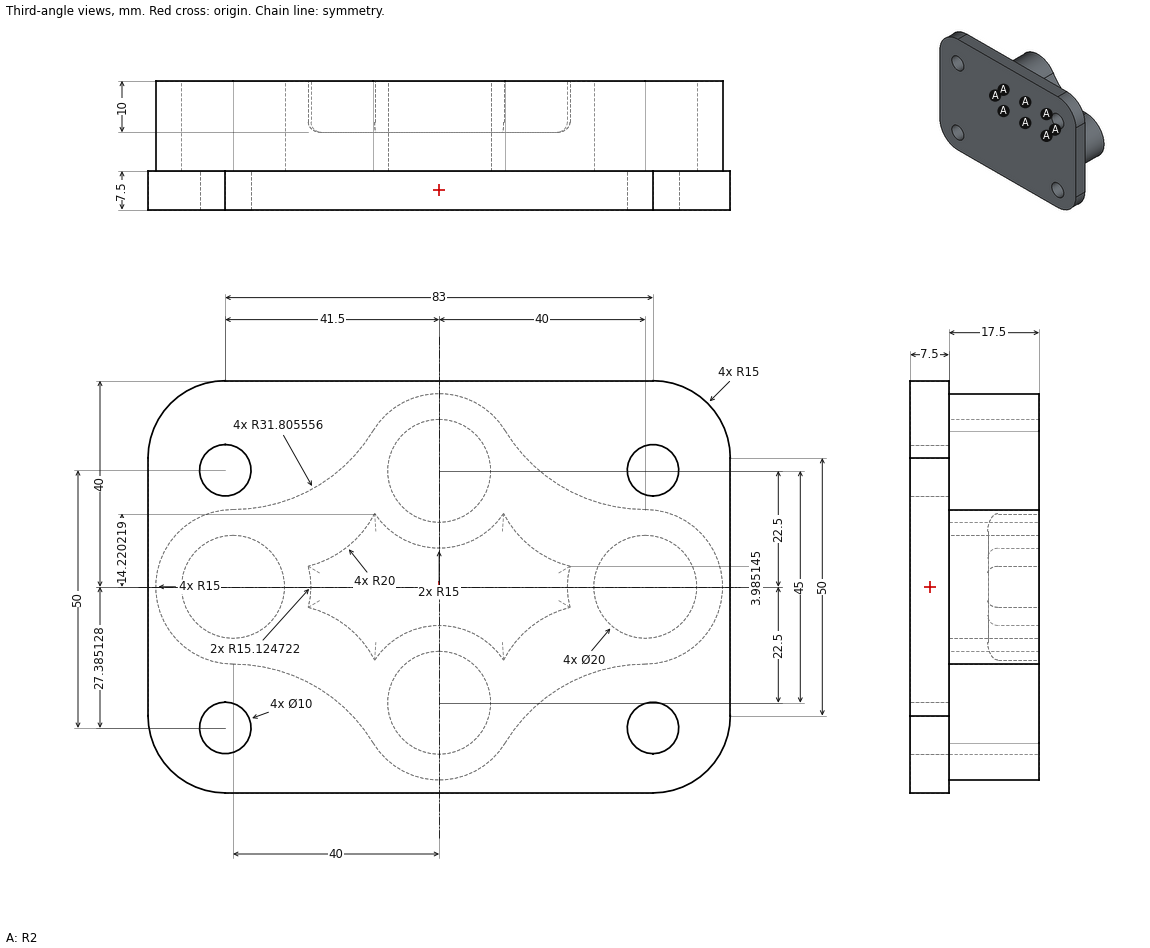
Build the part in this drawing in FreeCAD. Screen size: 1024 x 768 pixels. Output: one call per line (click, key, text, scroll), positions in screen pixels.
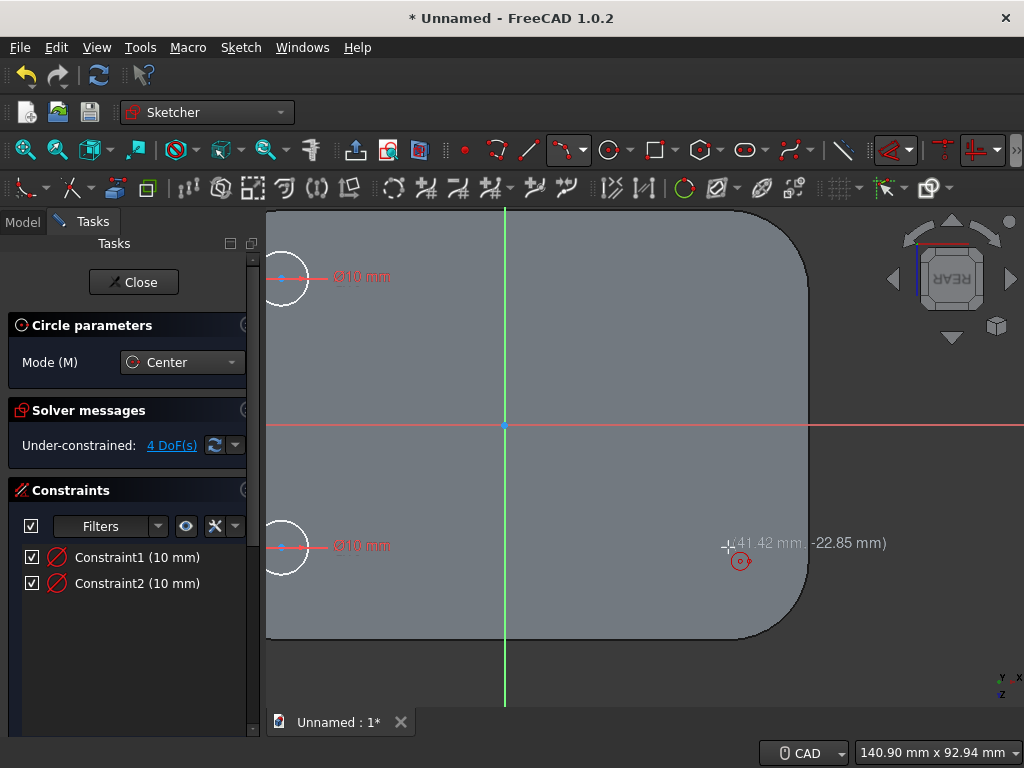
click(728, 547)
move(747, 528)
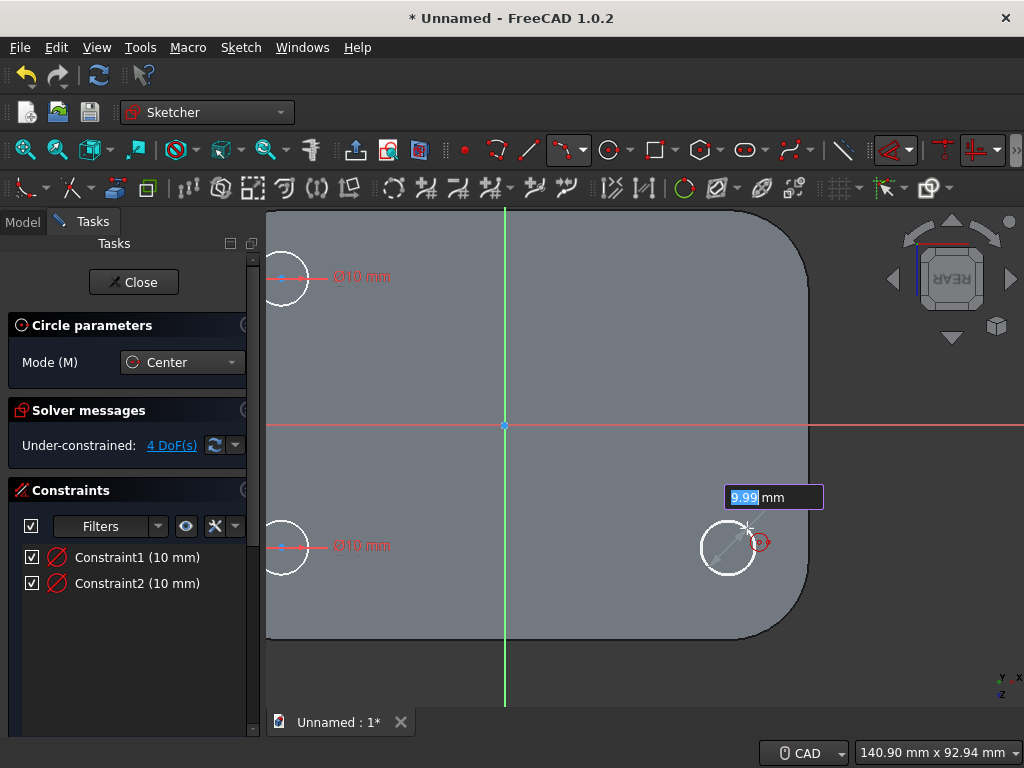
text(10)
key(Return)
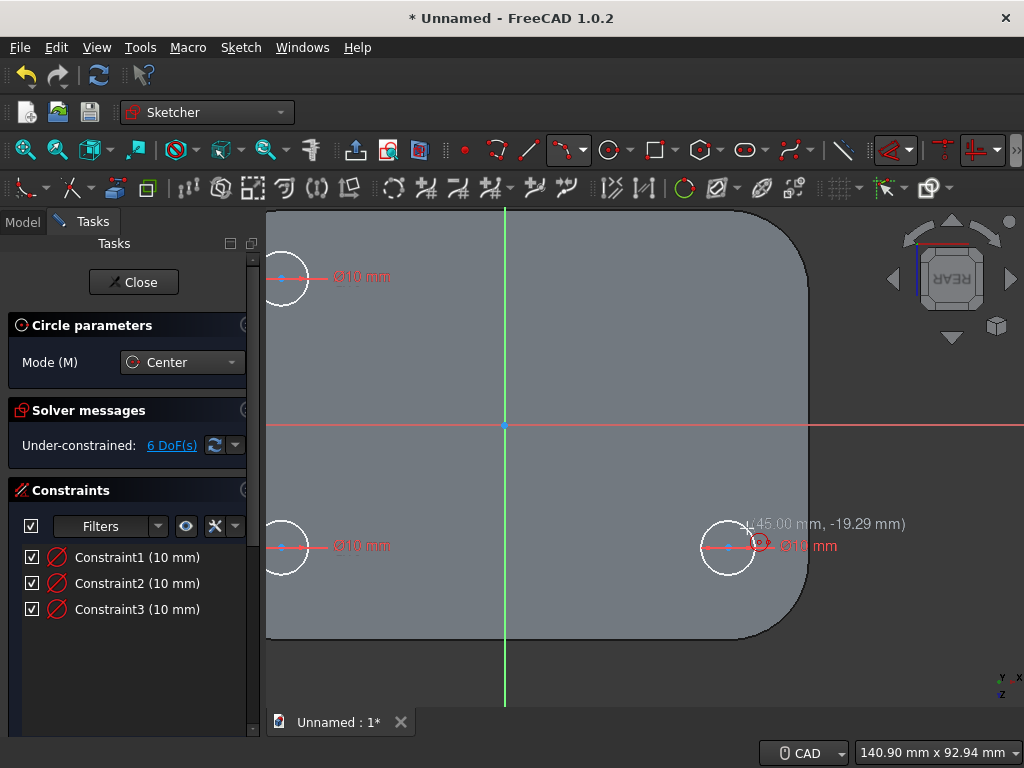
click(728, 278)
move(747, 259)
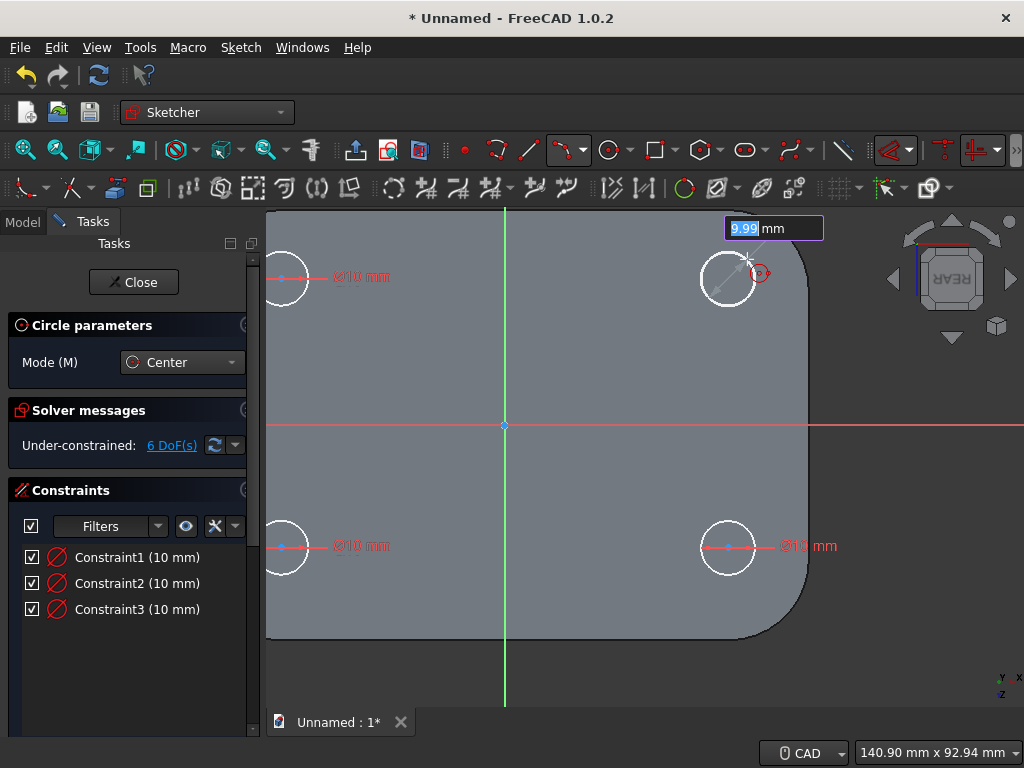
text(10)
key(Return)
key(Escape)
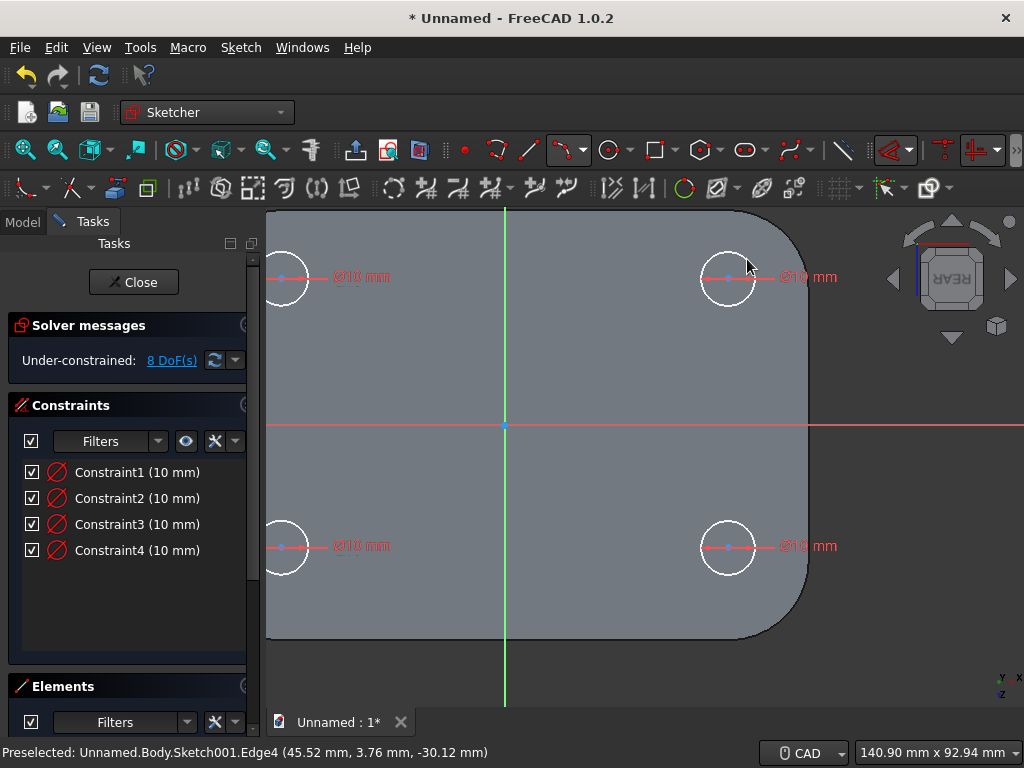
scroll(859, 659, down, 1)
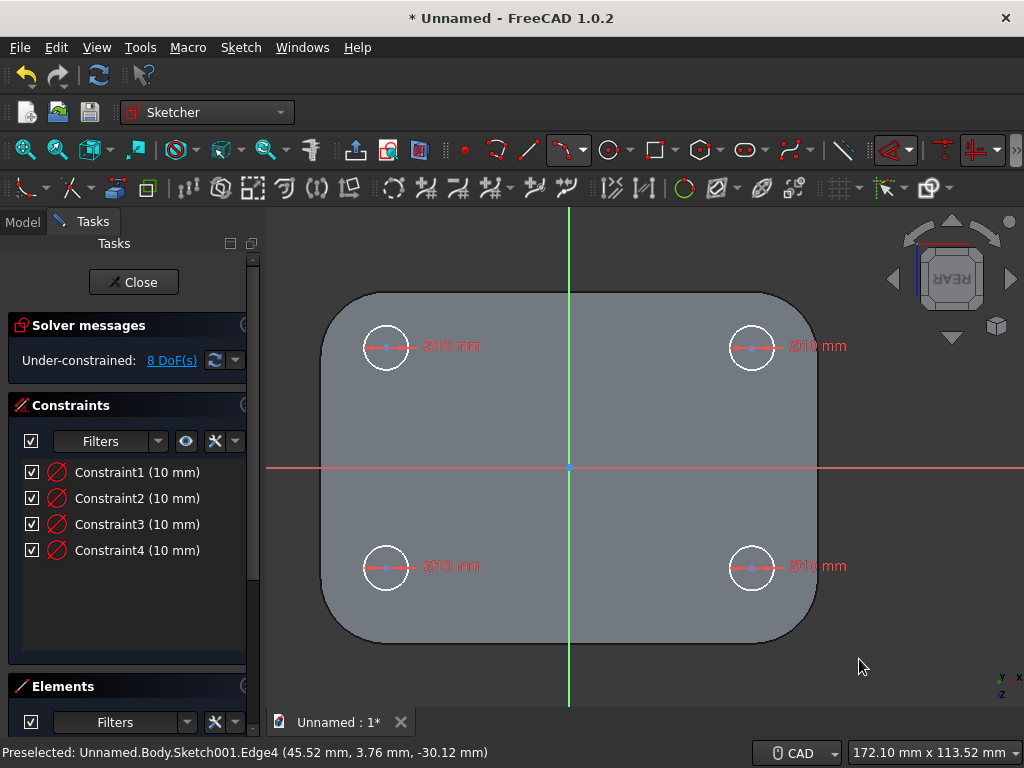
click(386, 348)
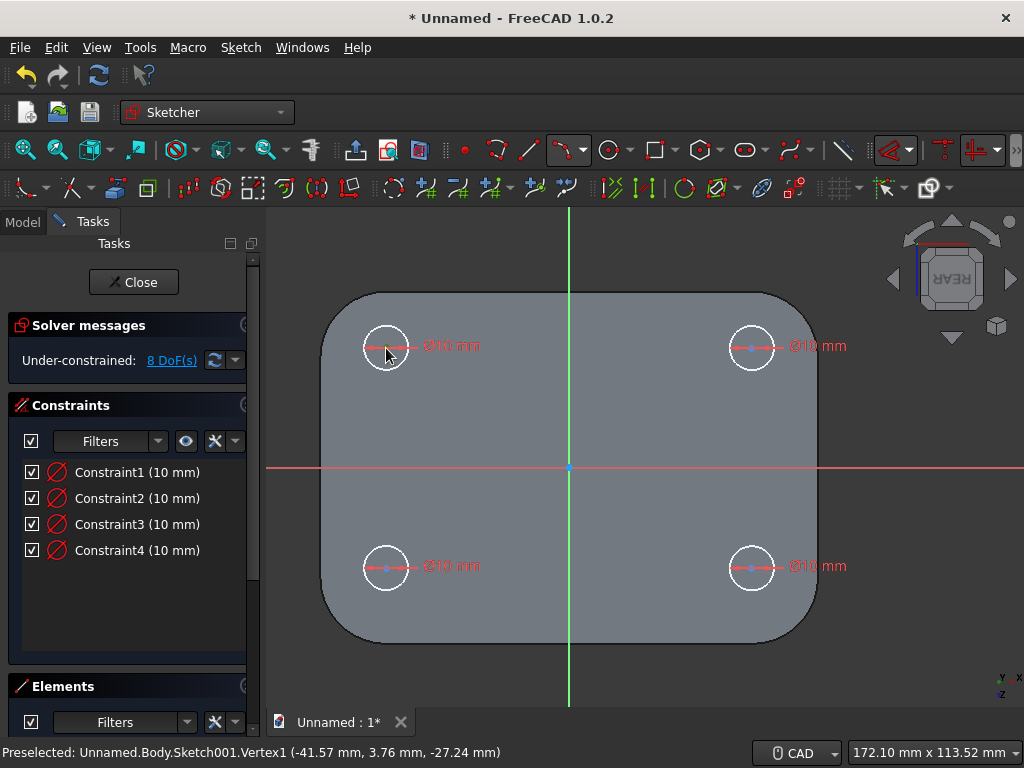
click(386, 568)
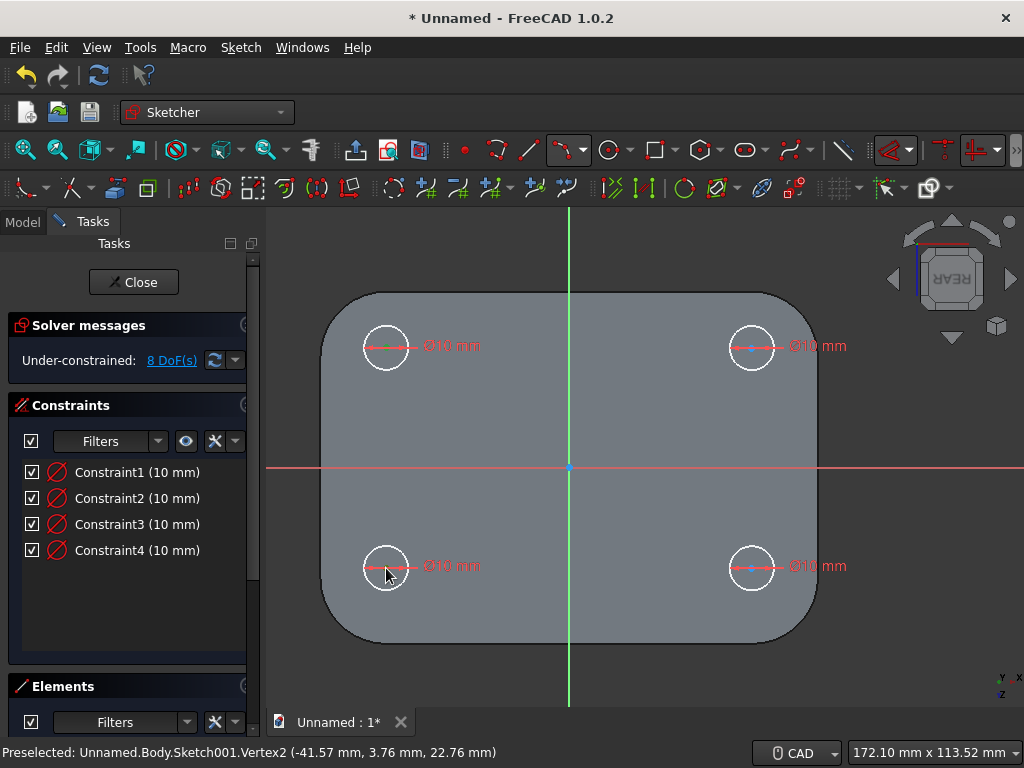
key(v)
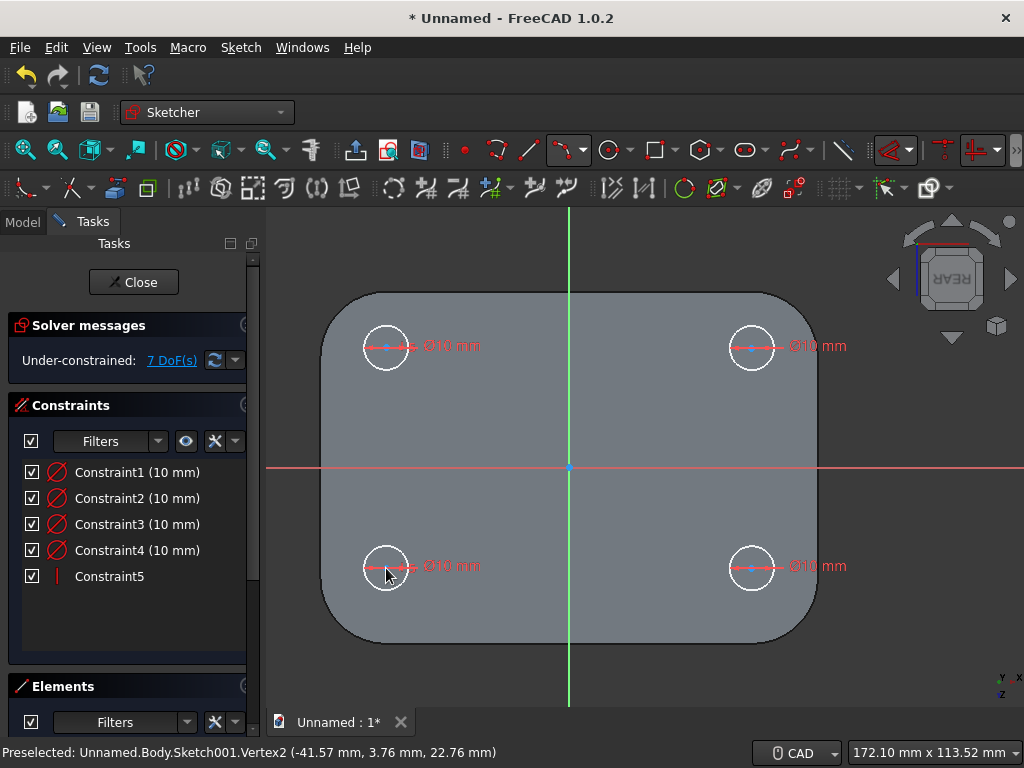
click(386, 568)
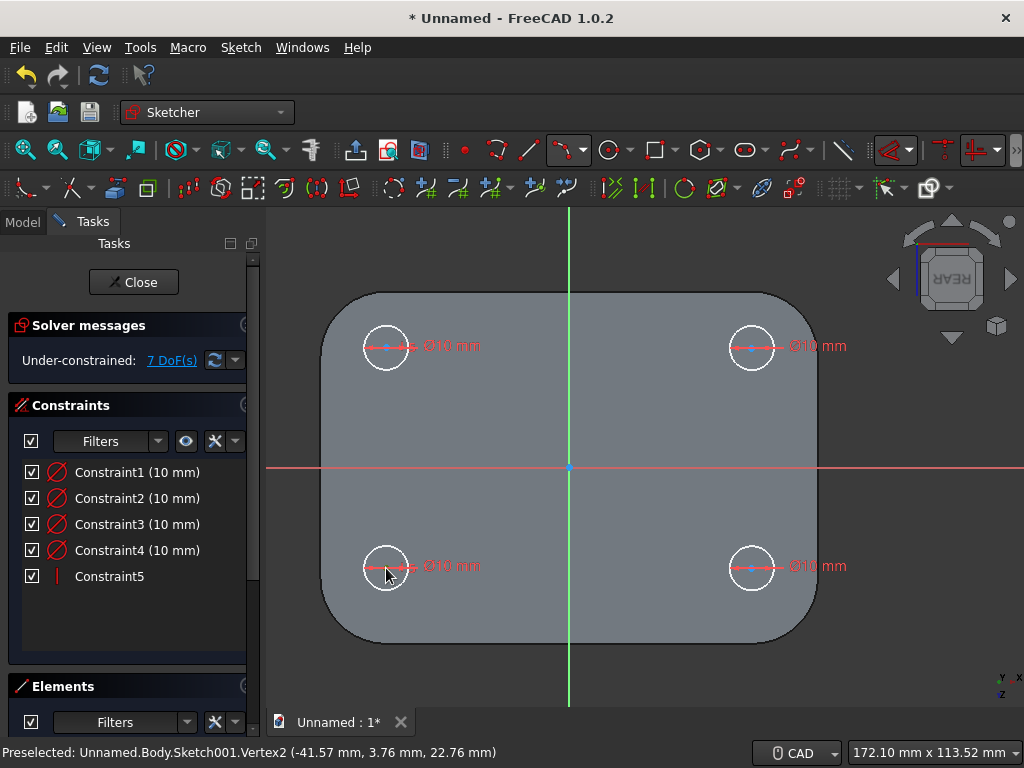
click(752, 568)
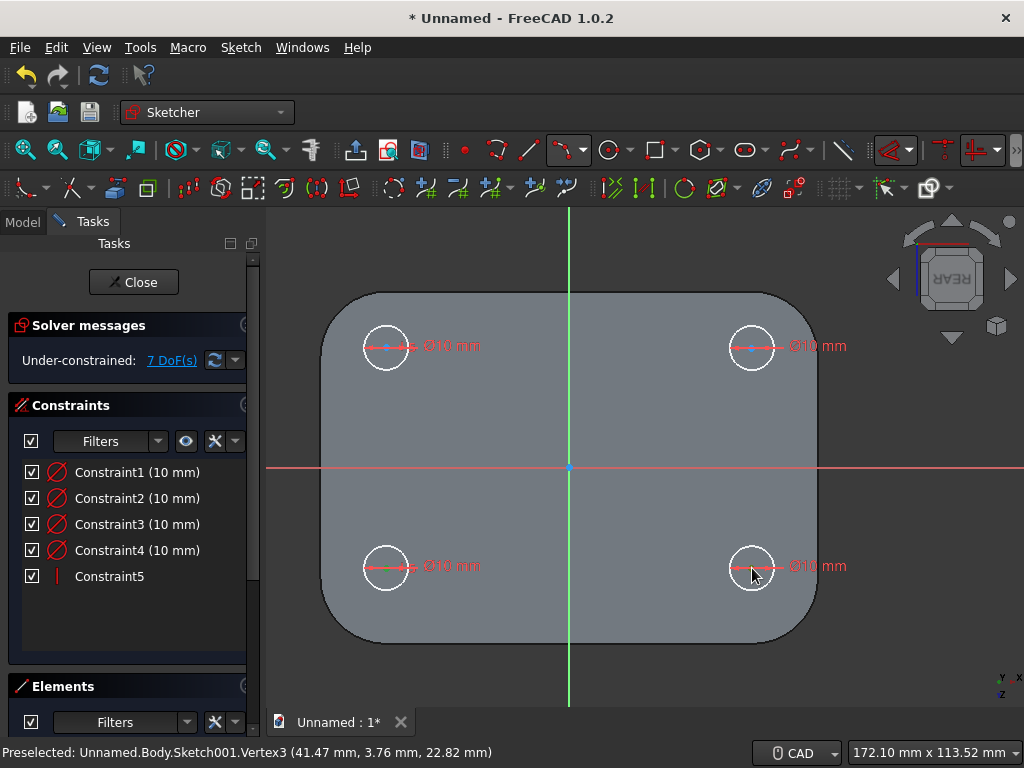
click(1000, 150)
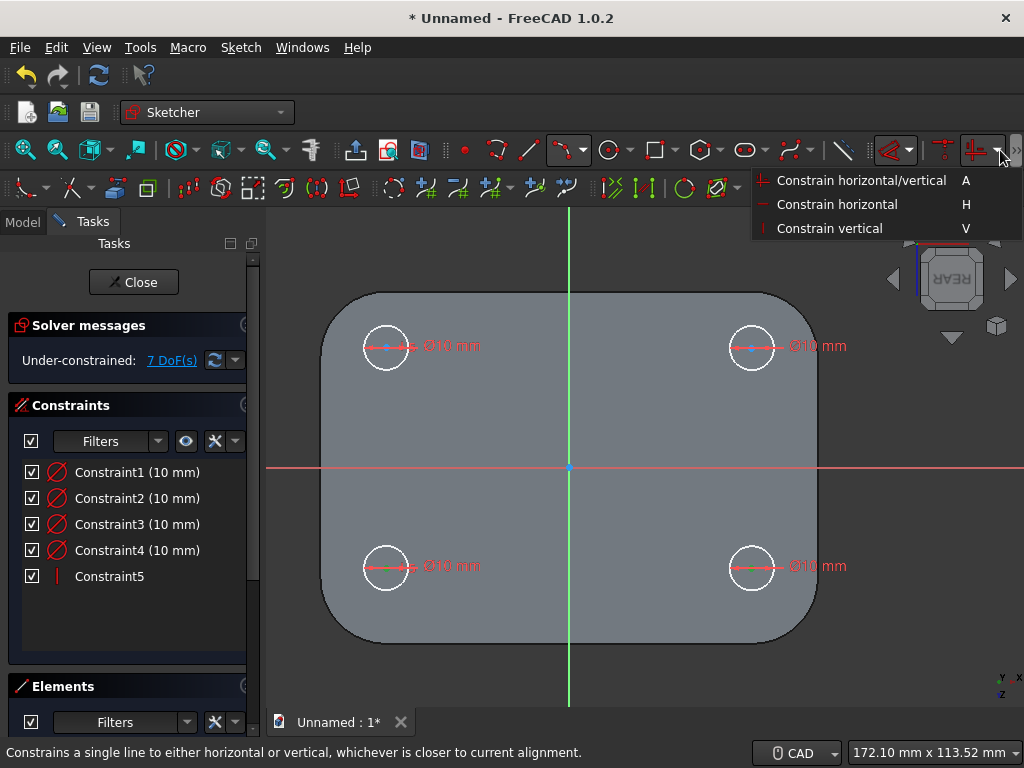
click(887, 204)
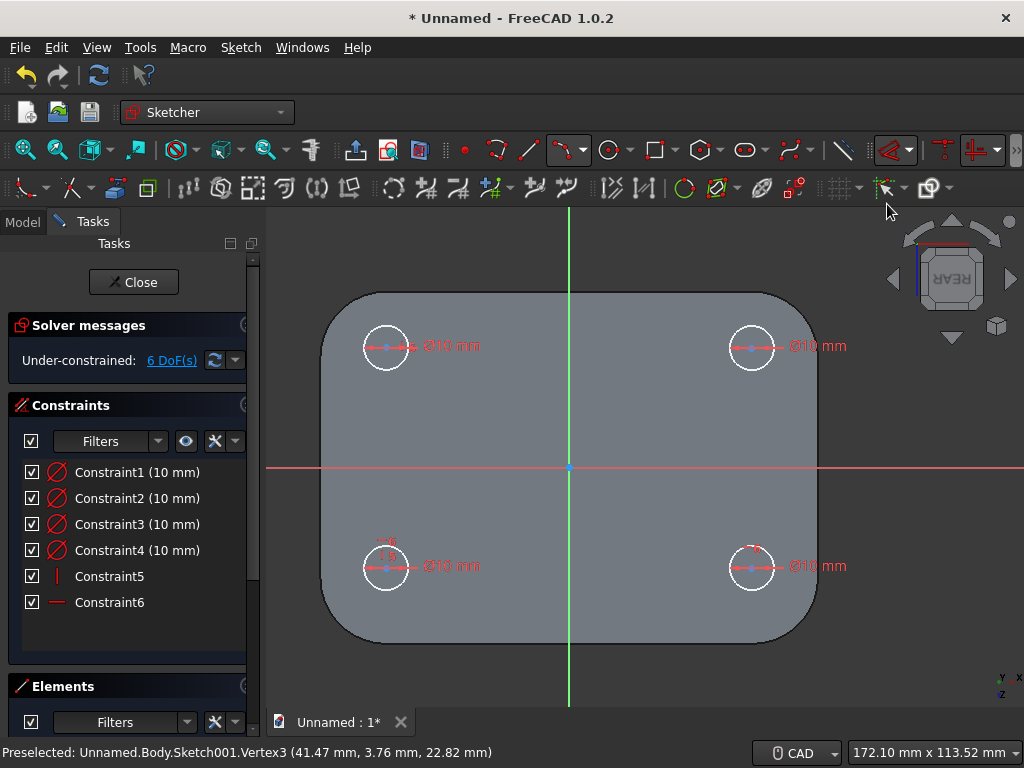
click(752, 568)